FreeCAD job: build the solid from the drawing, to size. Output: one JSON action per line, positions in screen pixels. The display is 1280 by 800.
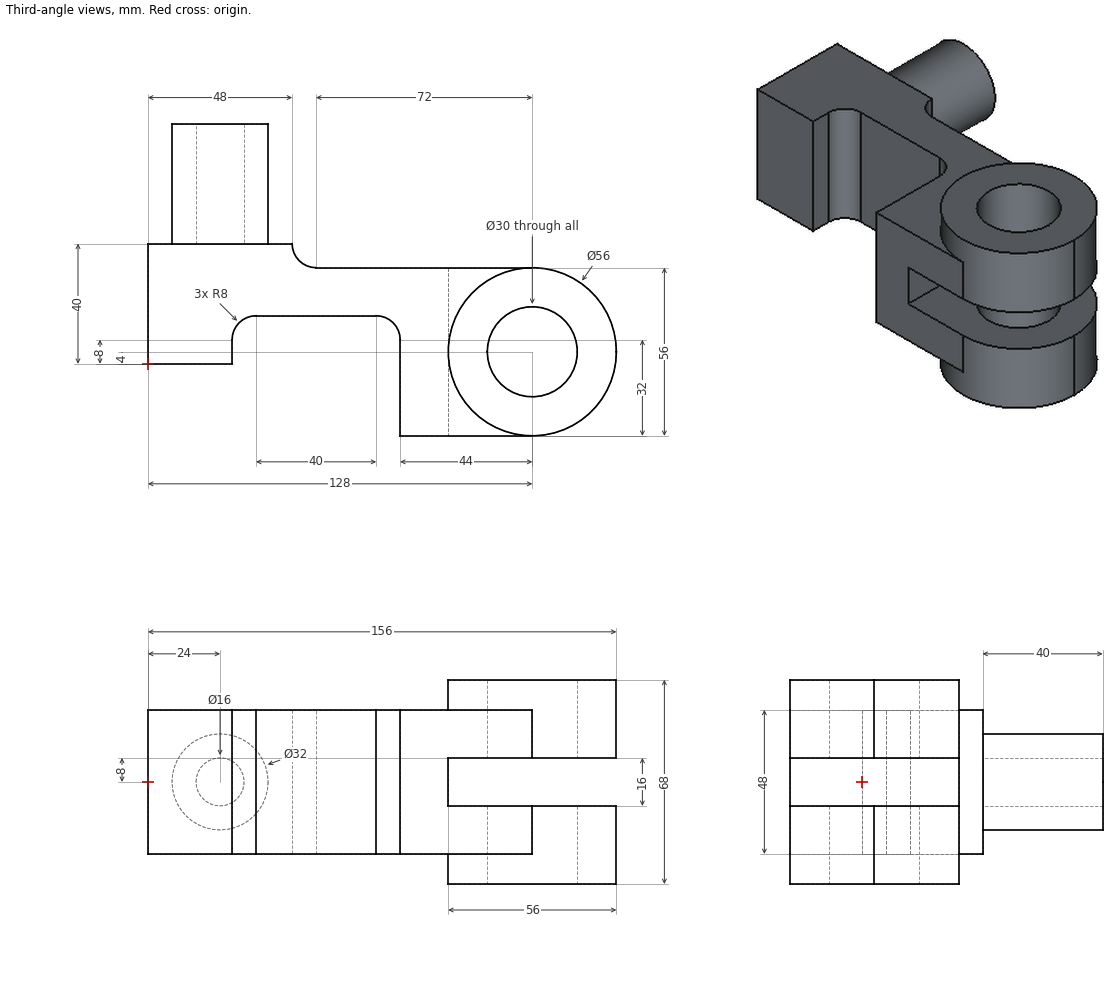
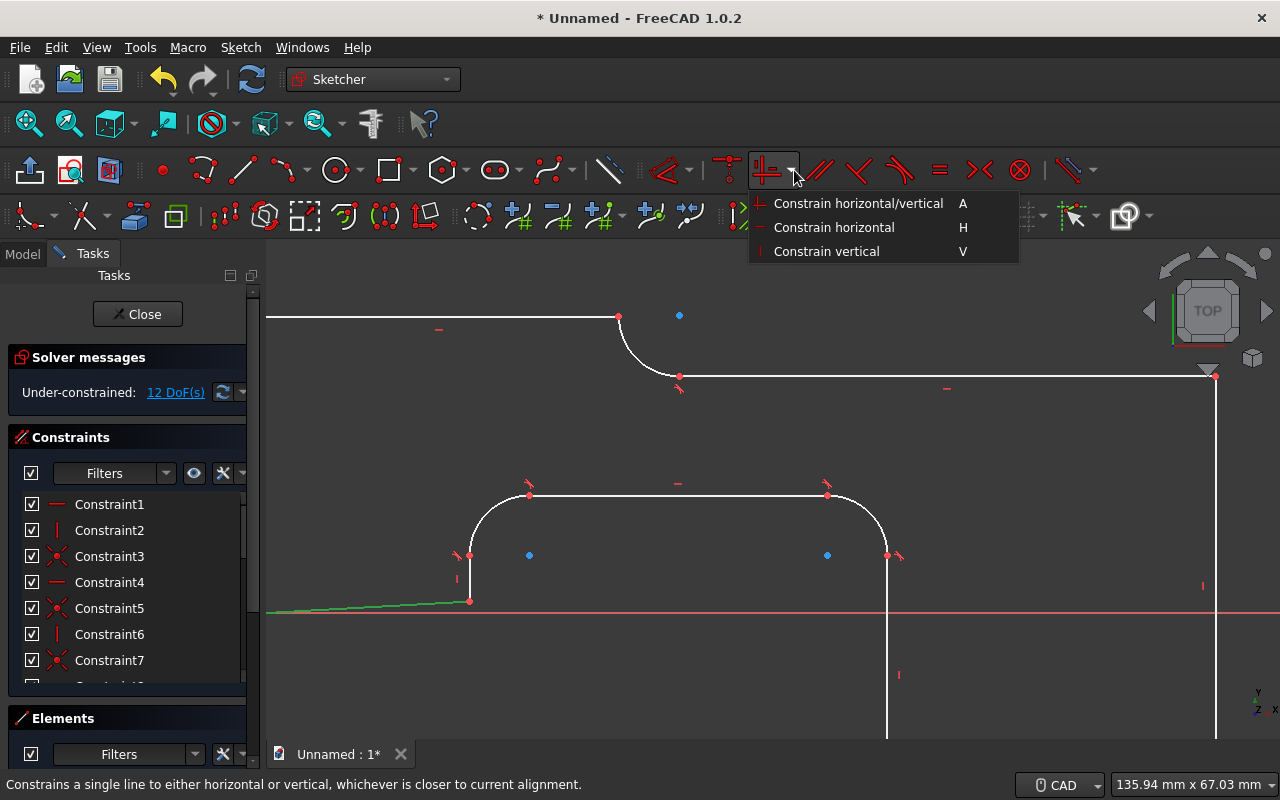
{"action": "left_click", "coordinate": [884, 227]}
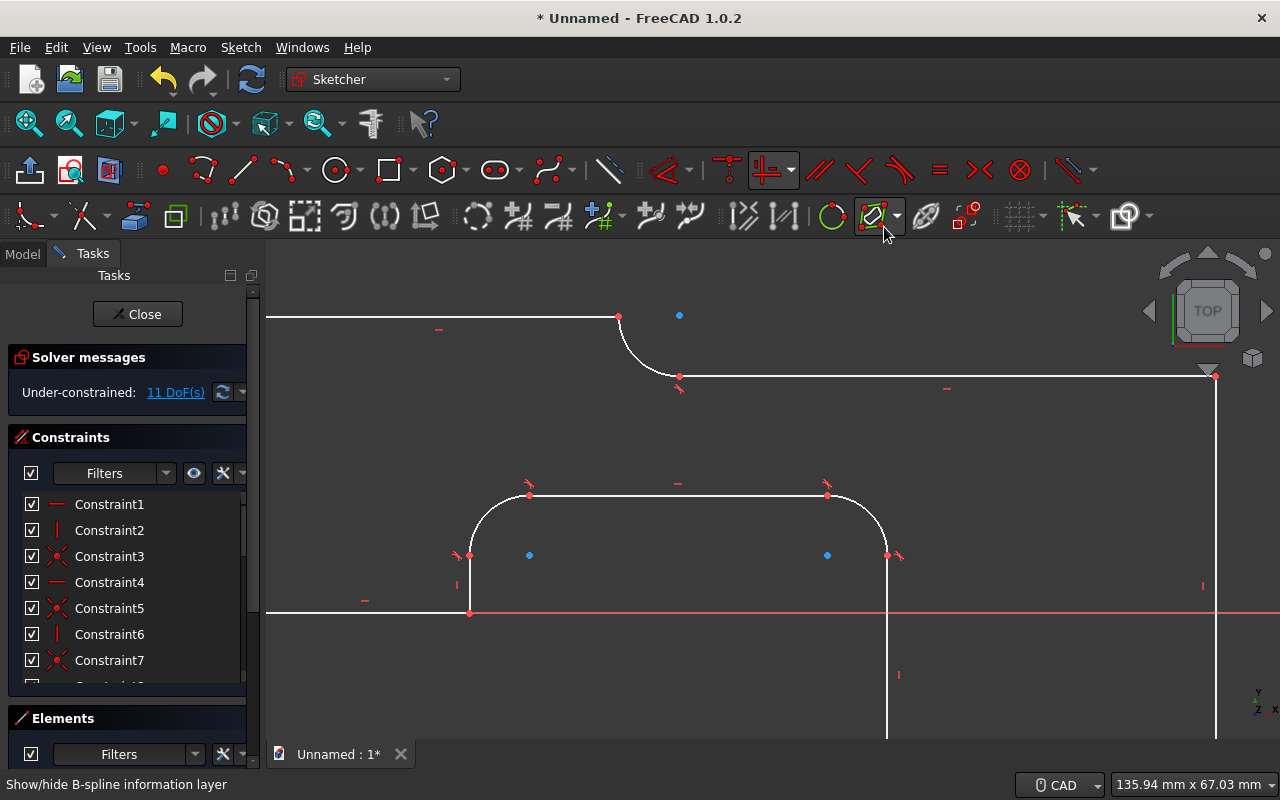
{"action": "left_click", "coordinate": [881, 528]}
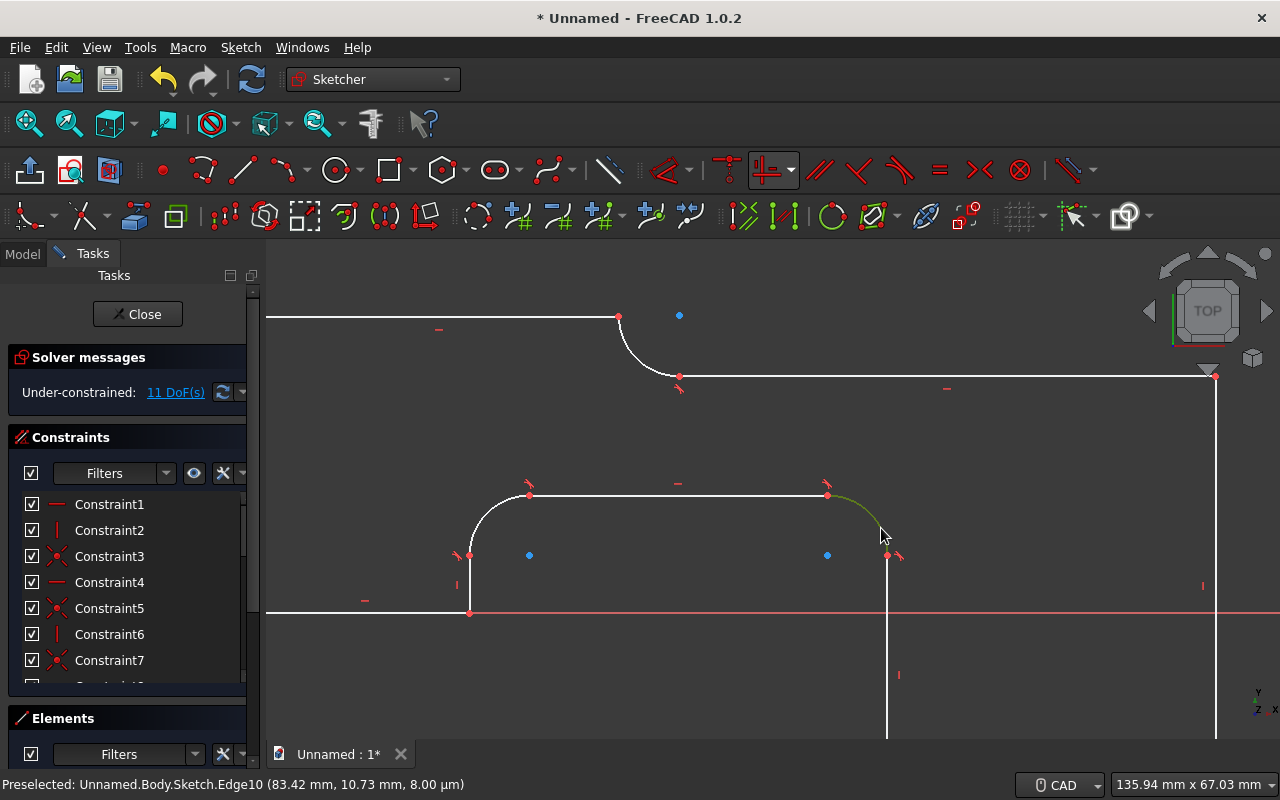
{"action": "left_click", "coordinate": [626, 344]}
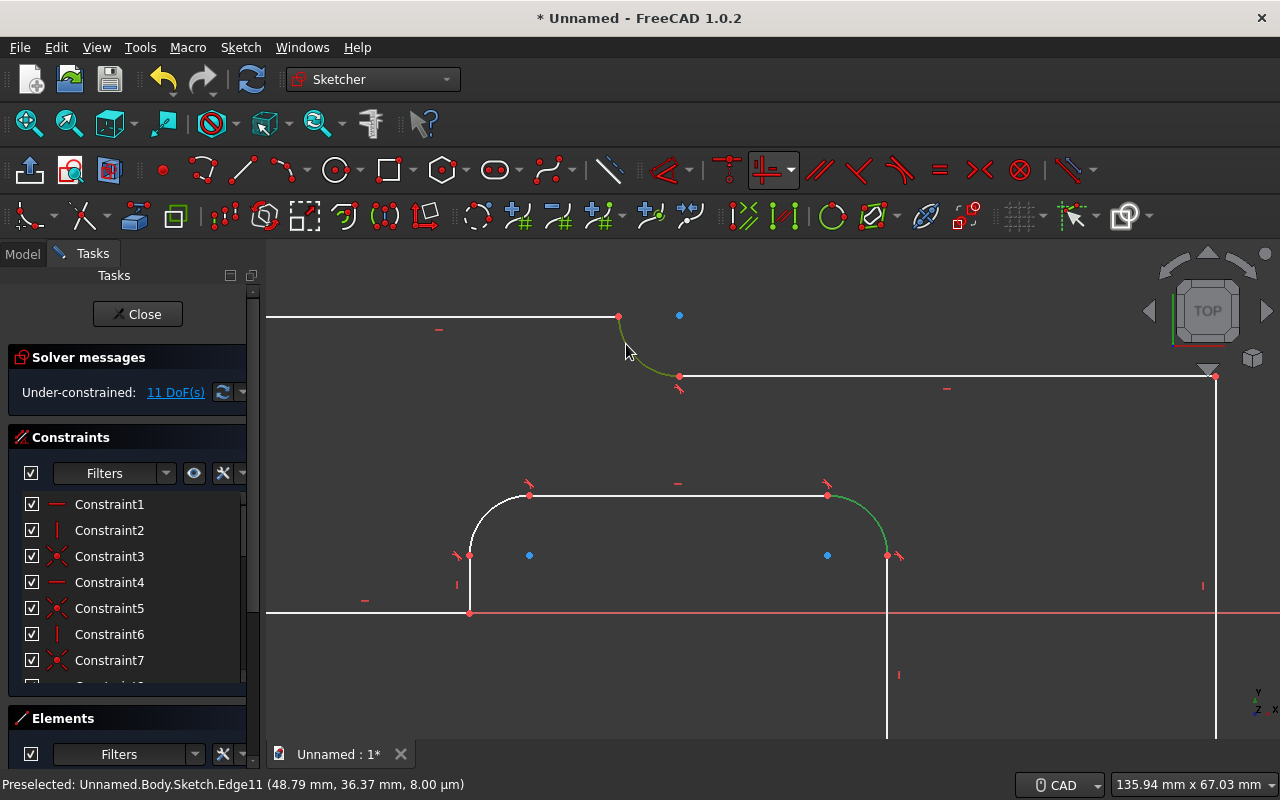
{"action": "left_click", "coordinate": [502, 502]}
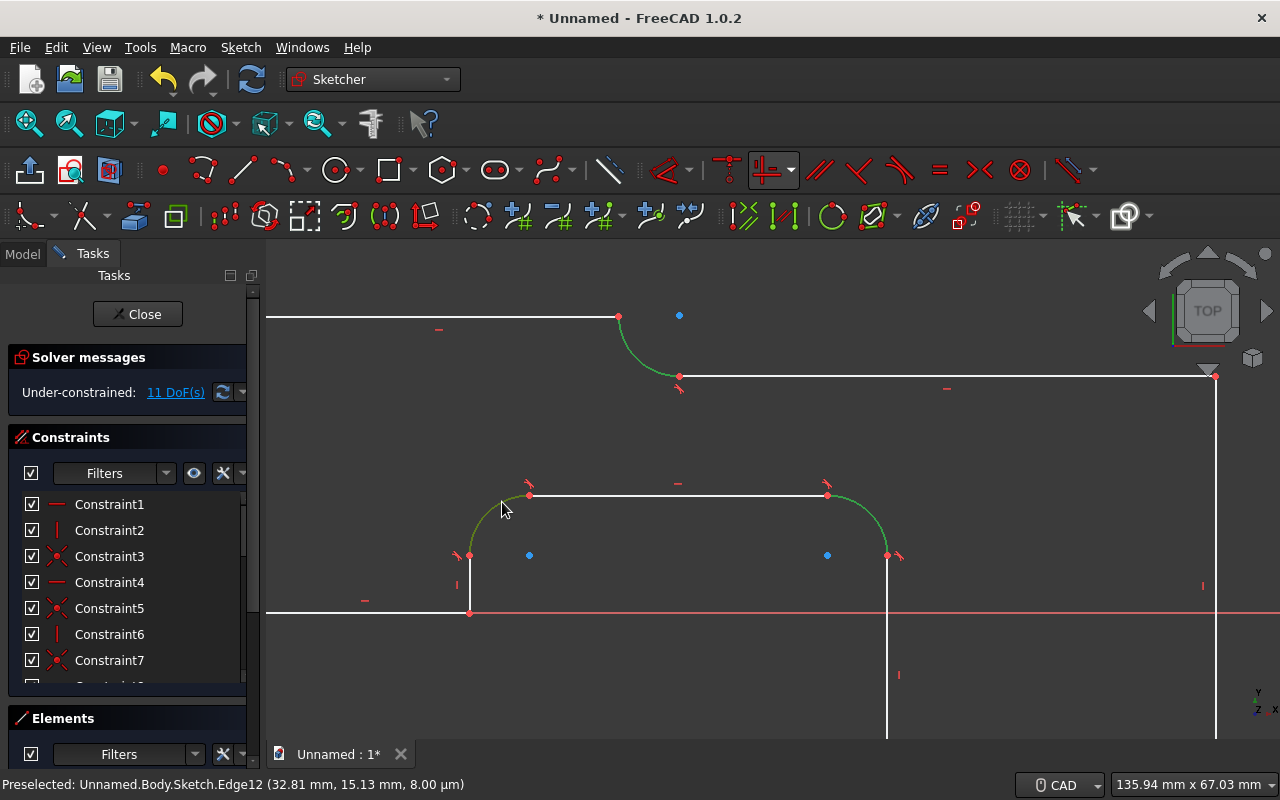
{"action": "left_click", "coordinate": [940, 170]}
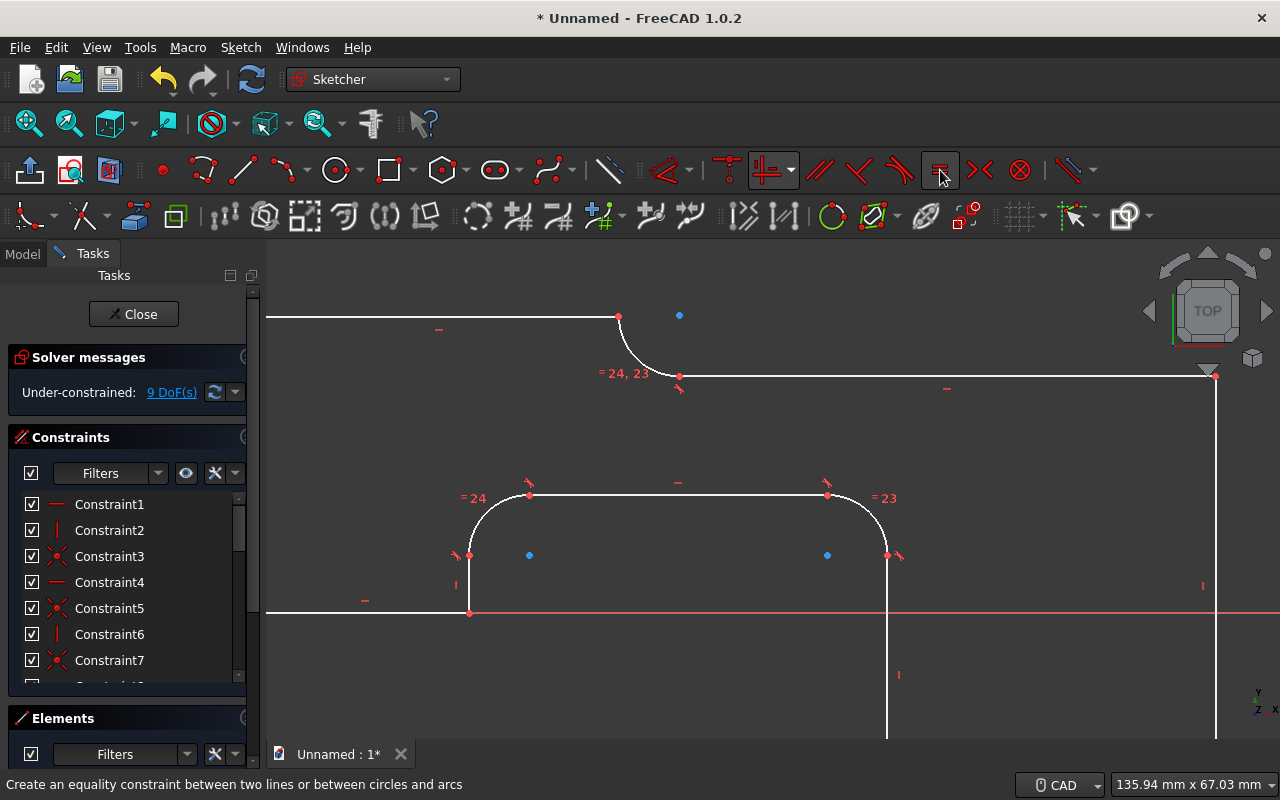
{"action": "key", "text": "d"}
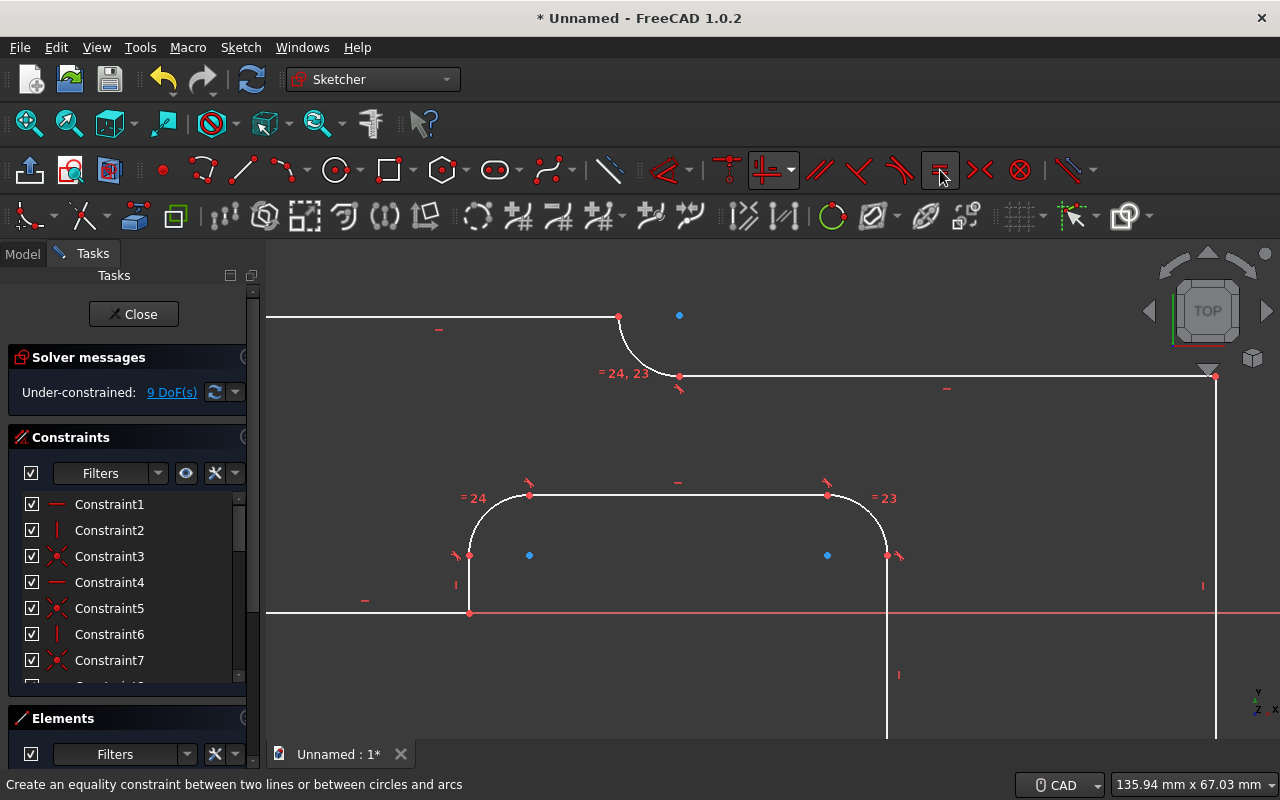
{"action": "left_click", "coordinate": [881, 528]}
{"action": "left_click", "coordinate": [910, 514]}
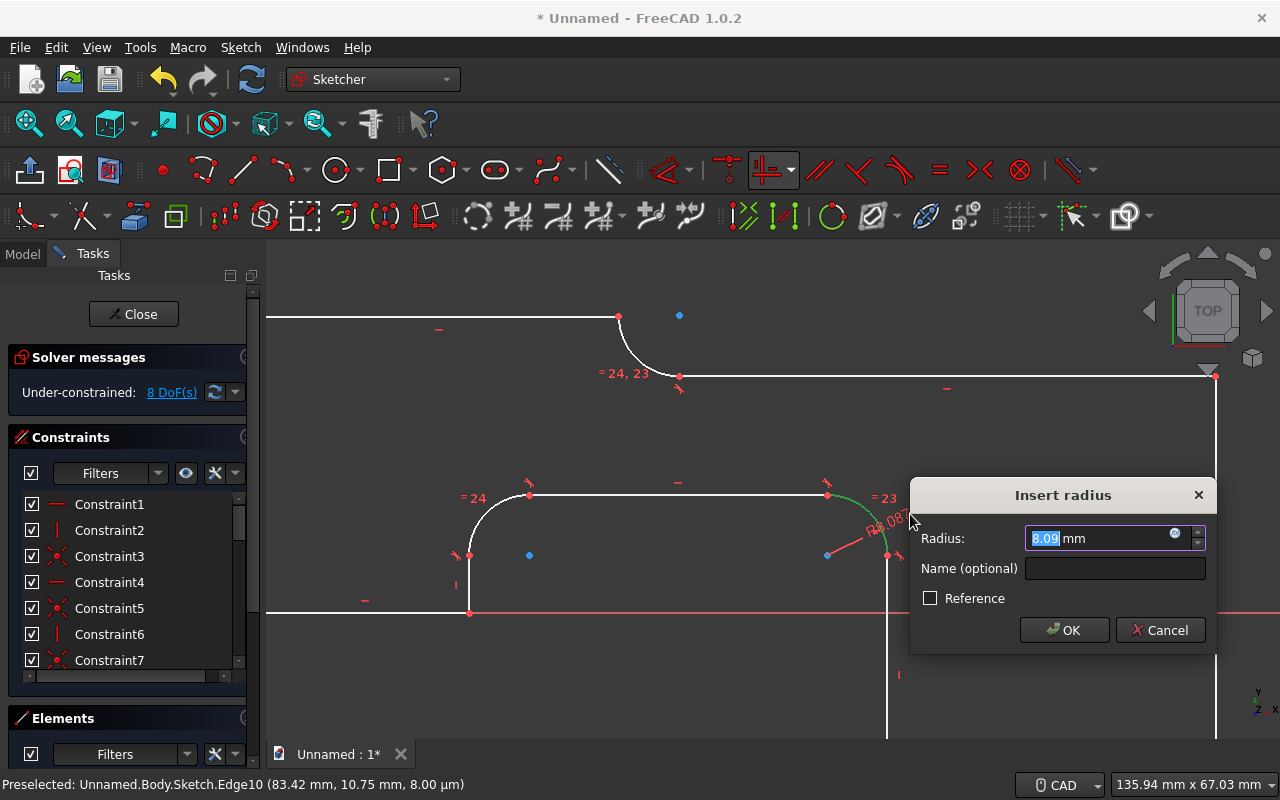
{"action": "type", "text": "8"}
{"action": "key", "text": "Return"}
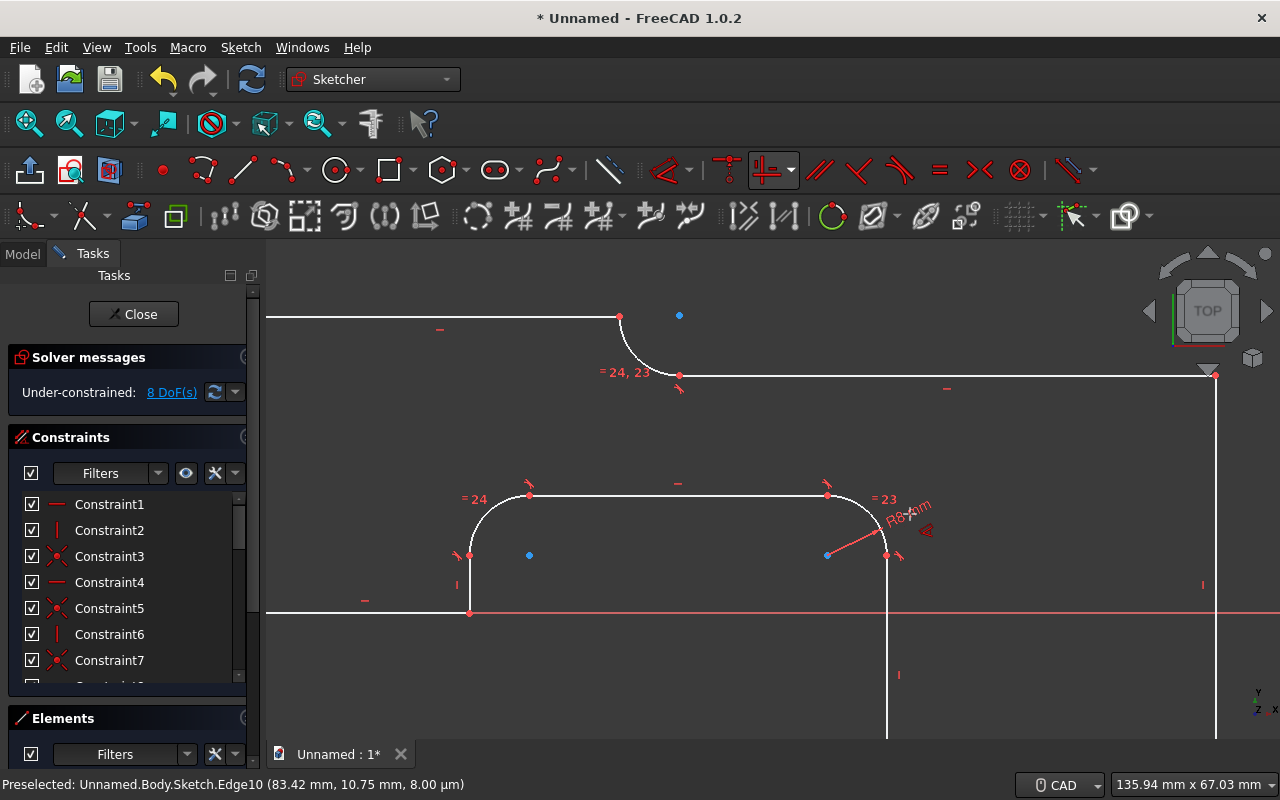
{"action": "left_click", "coordinate": [470, 596]}
{"action": "left_click", "coordinate": [436, 584]}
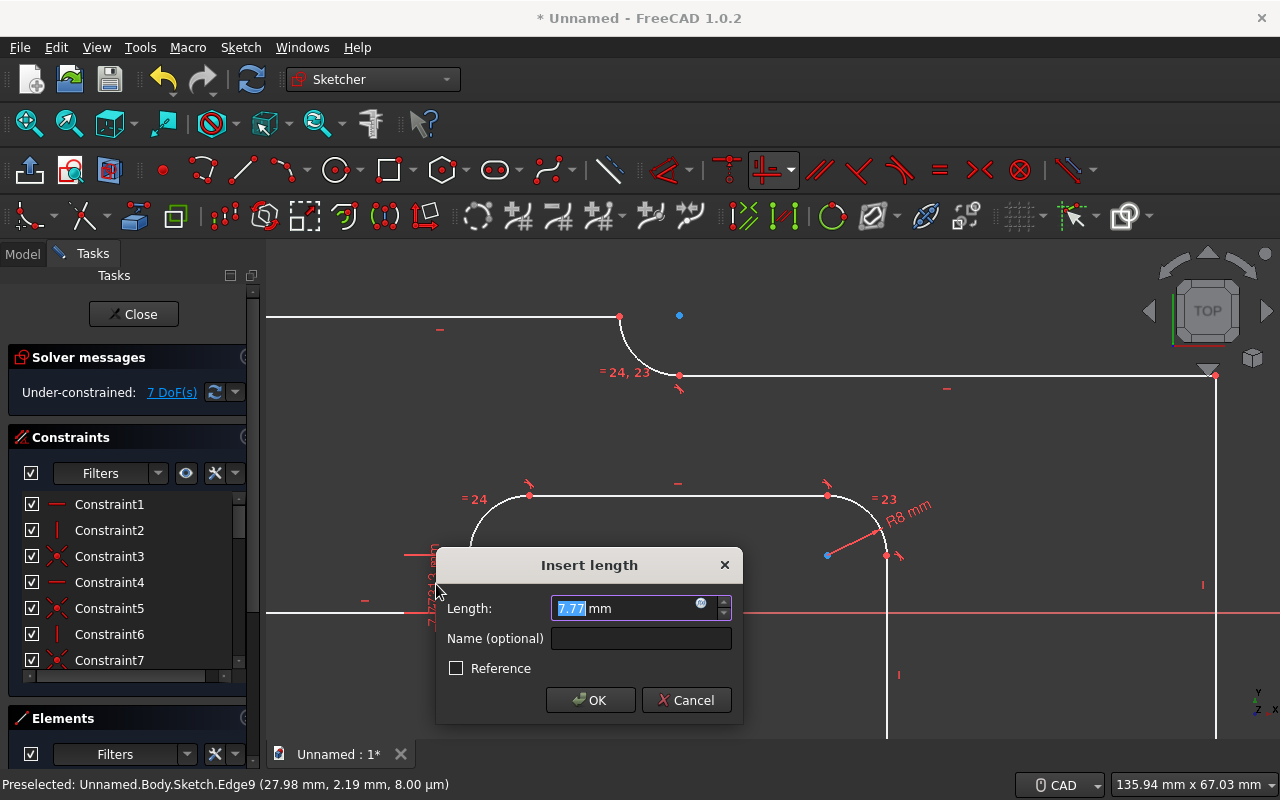
{"action": "type", "text": "8"}
{"action": "key", "text": "Return"}